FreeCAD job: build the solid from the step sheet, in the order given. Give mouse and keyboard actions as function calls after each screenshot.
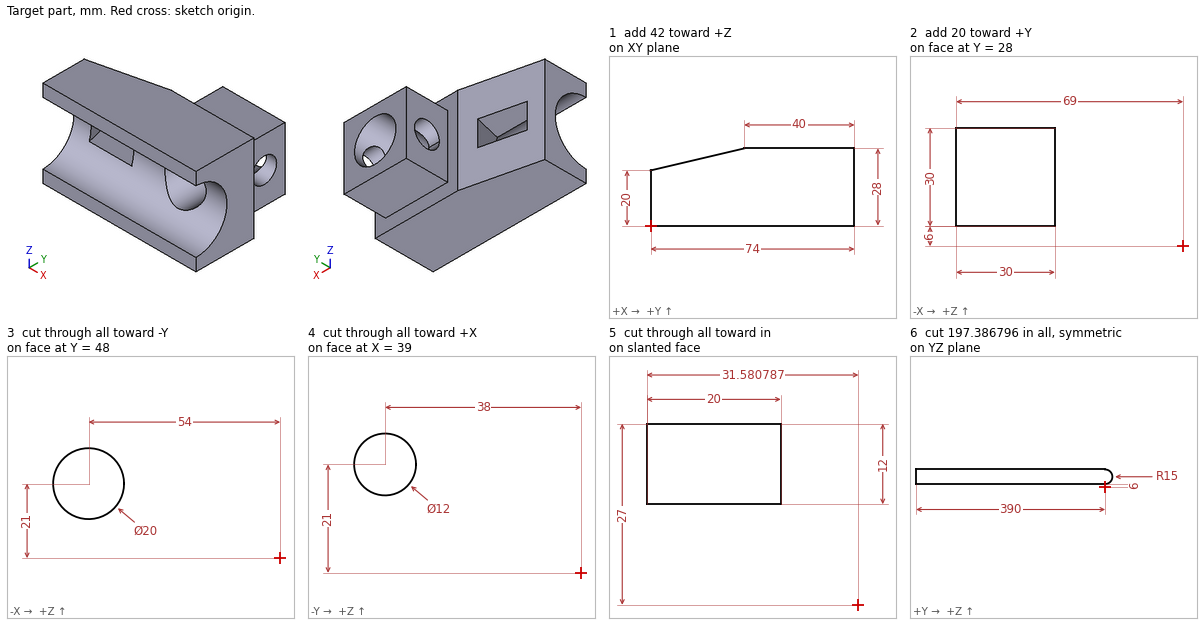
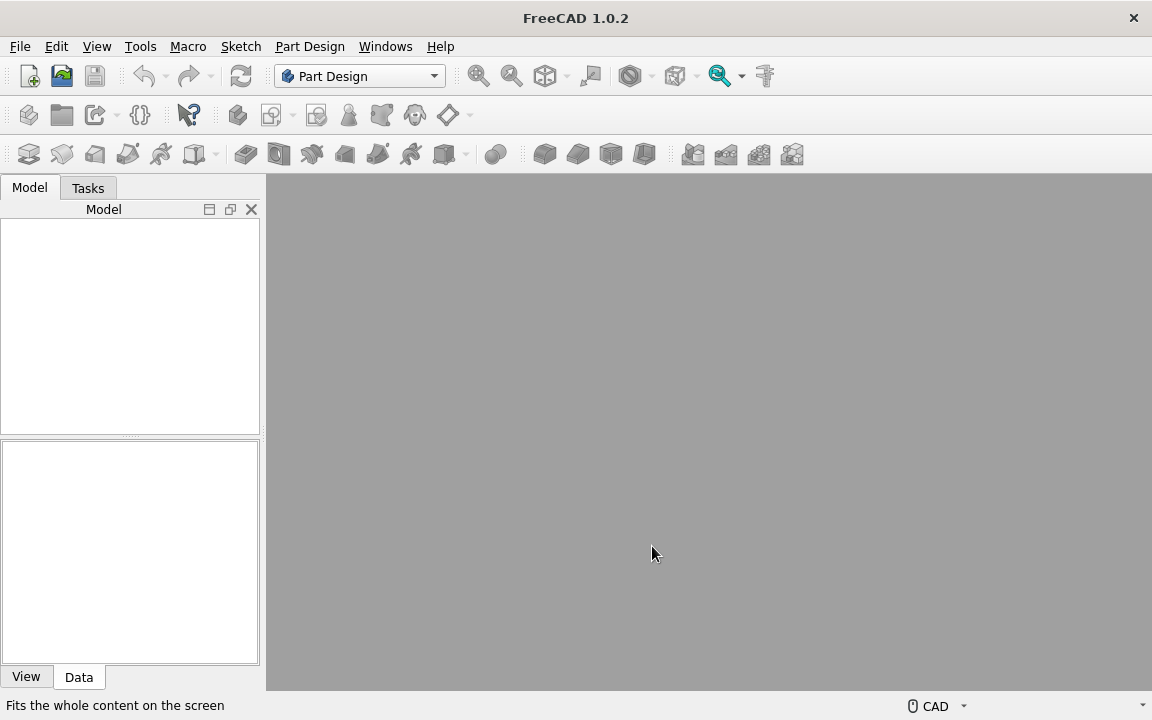
click(29, 76)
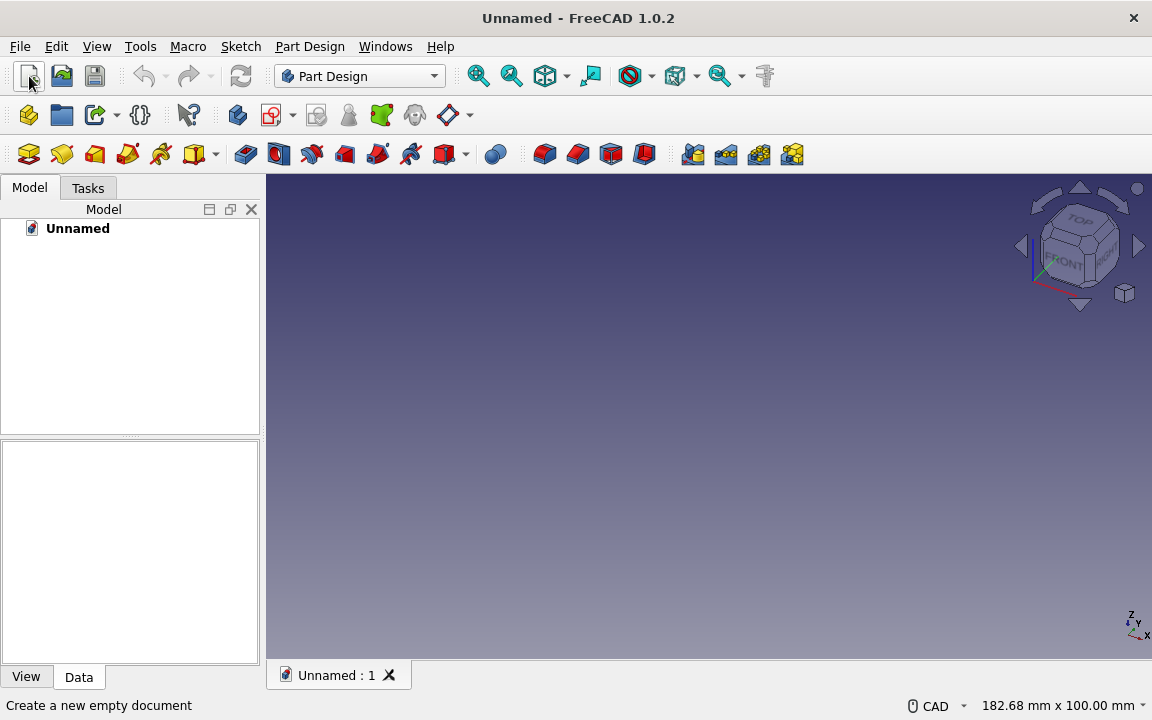
click(270, 116)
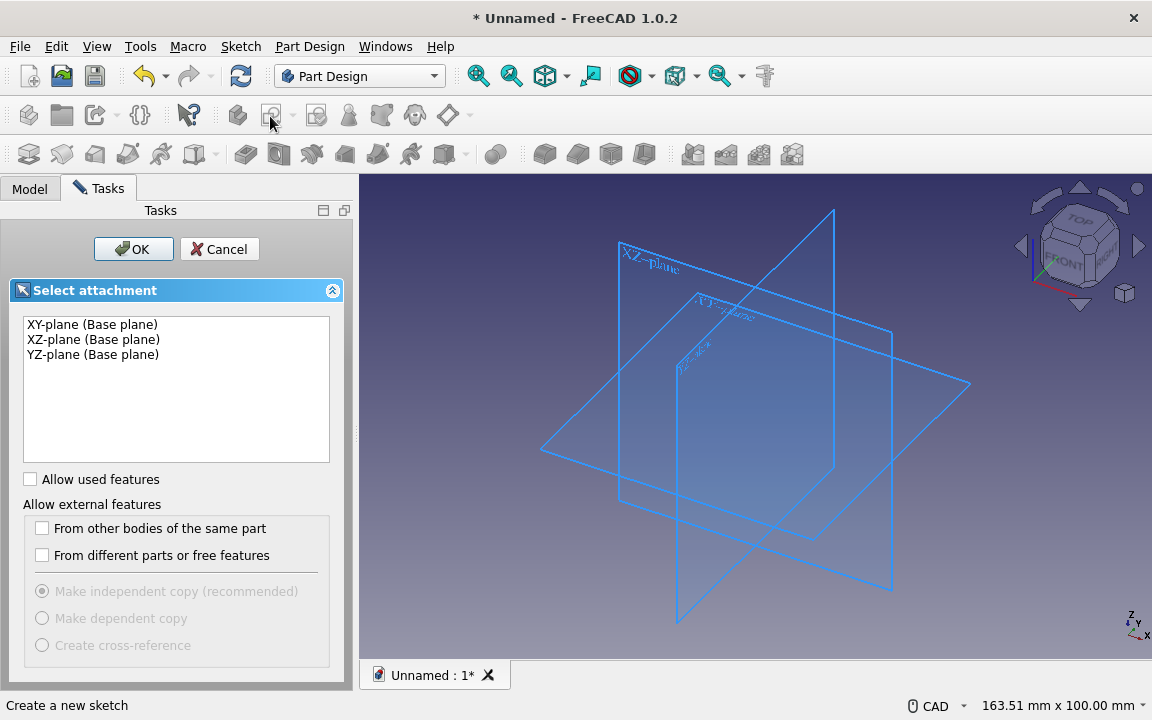
click(84, 324)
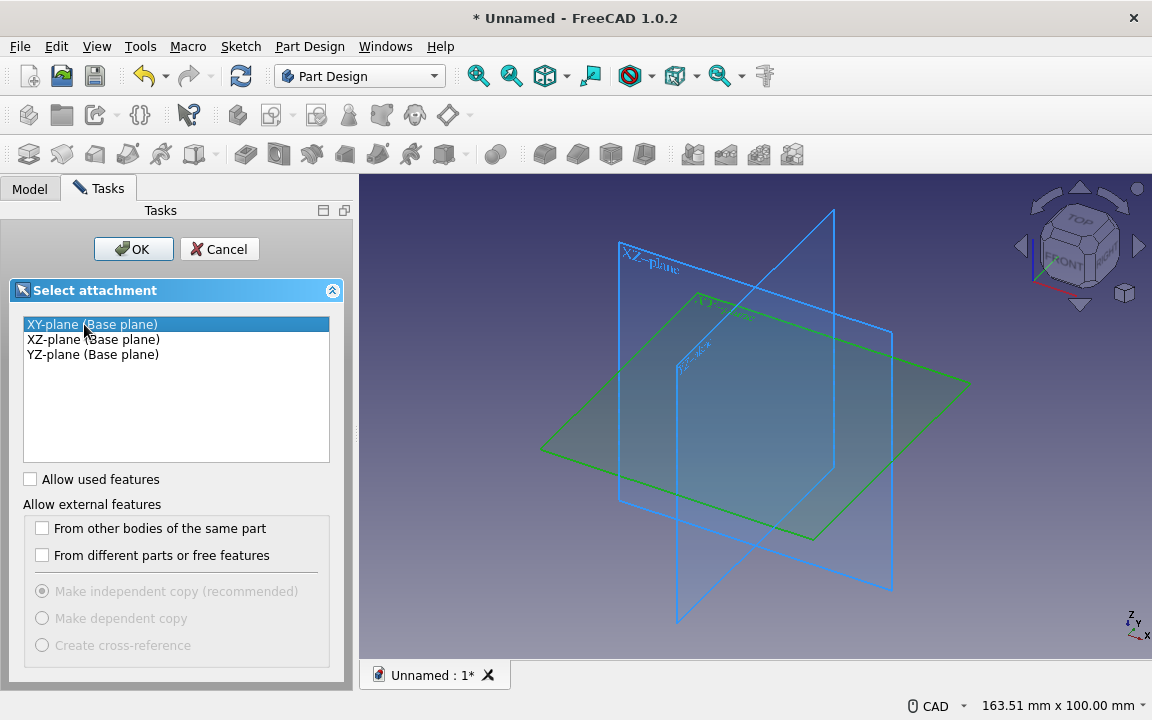
click(134, 249)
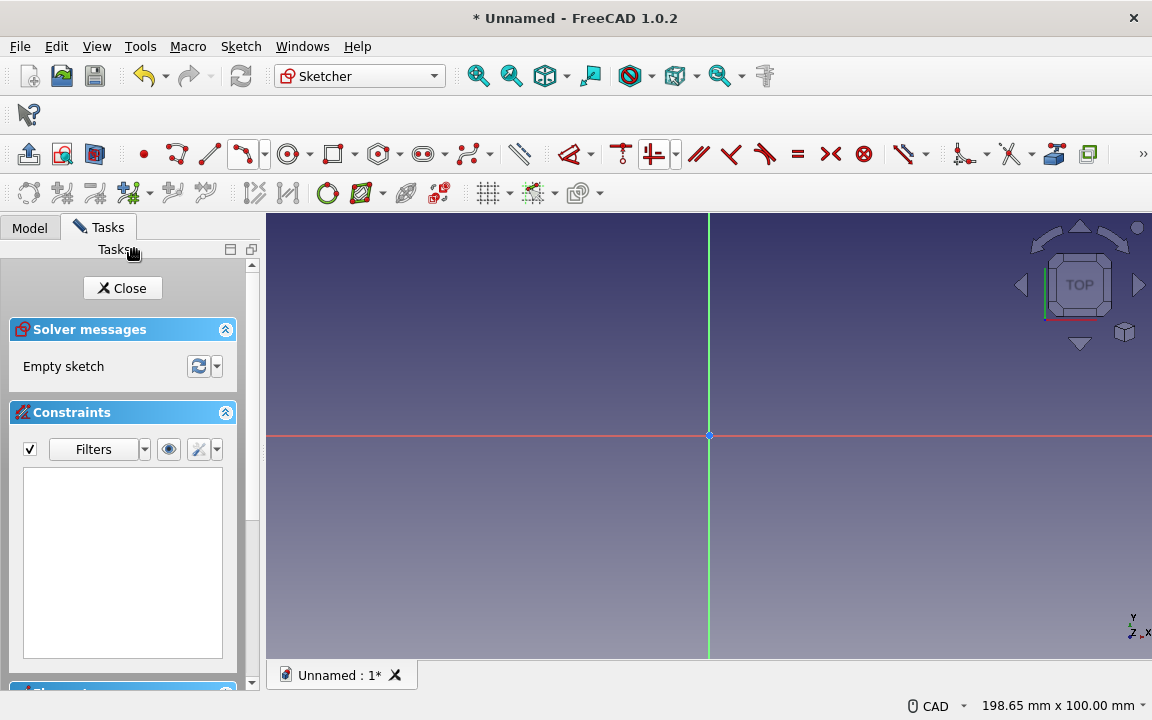
scroll(294, 631, down, 1)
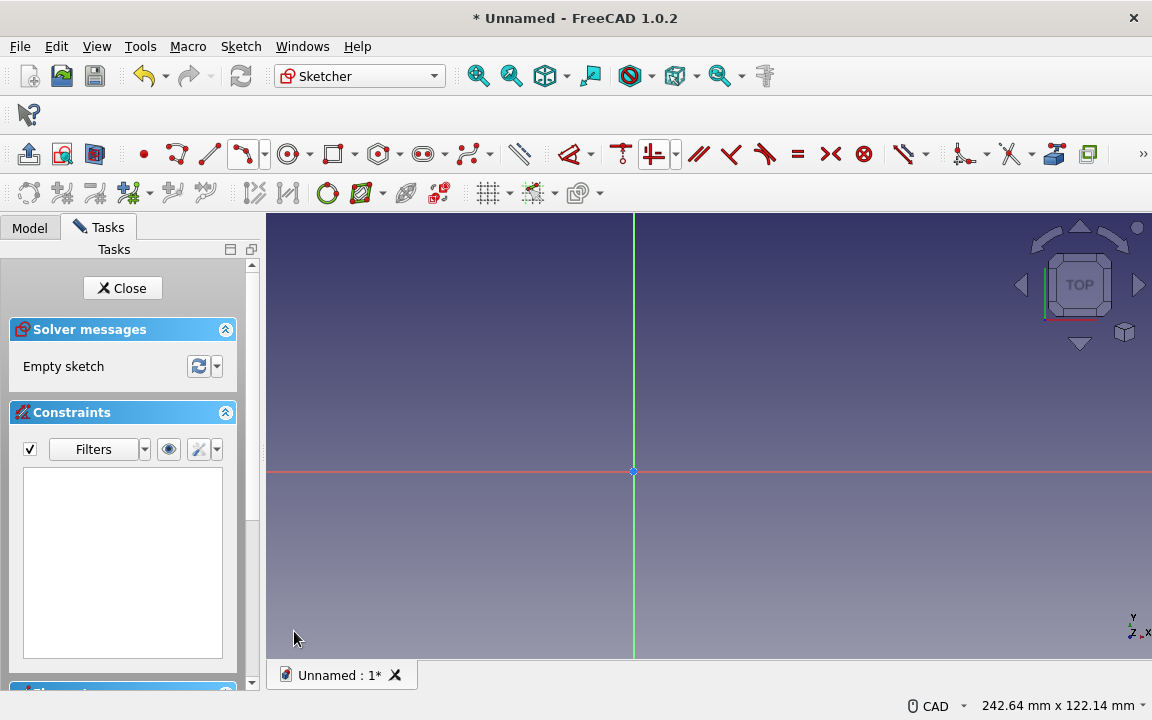
scroll(925, 401, up, 3)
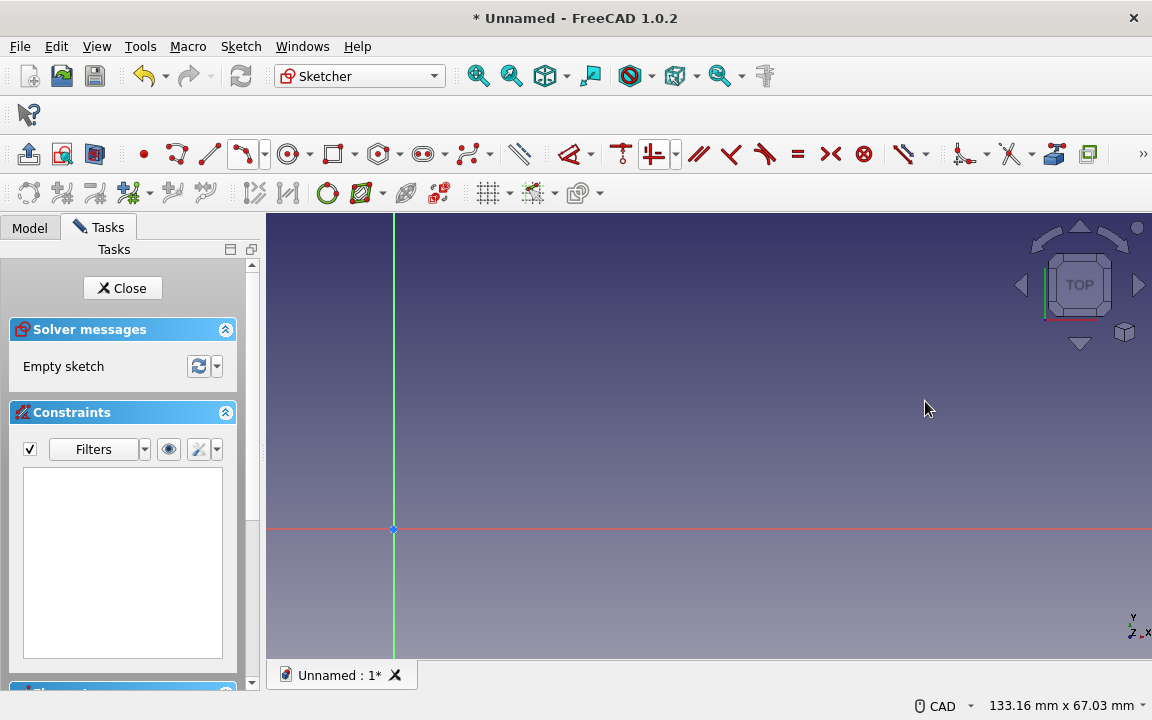
click(177, 154)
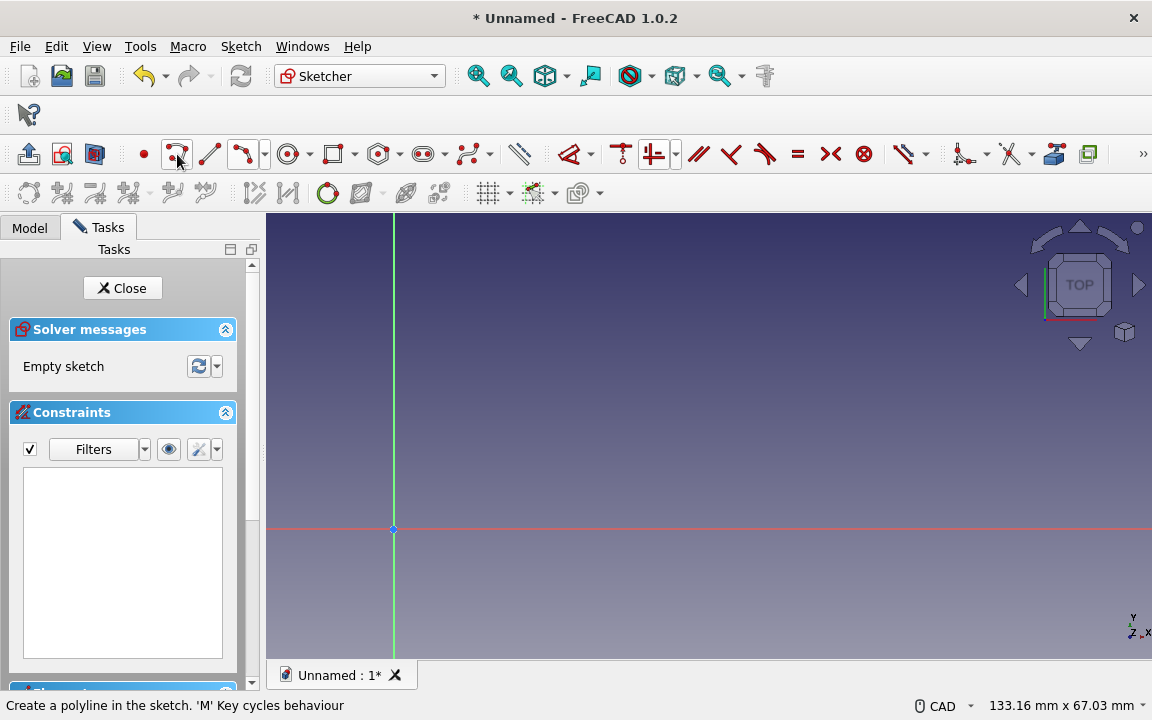
click(394, 529)
click(886, 520)
click(886, 343)
click(620, 343)
click(403, 396)
click(394, 529)
key(Escape)
key(Escape)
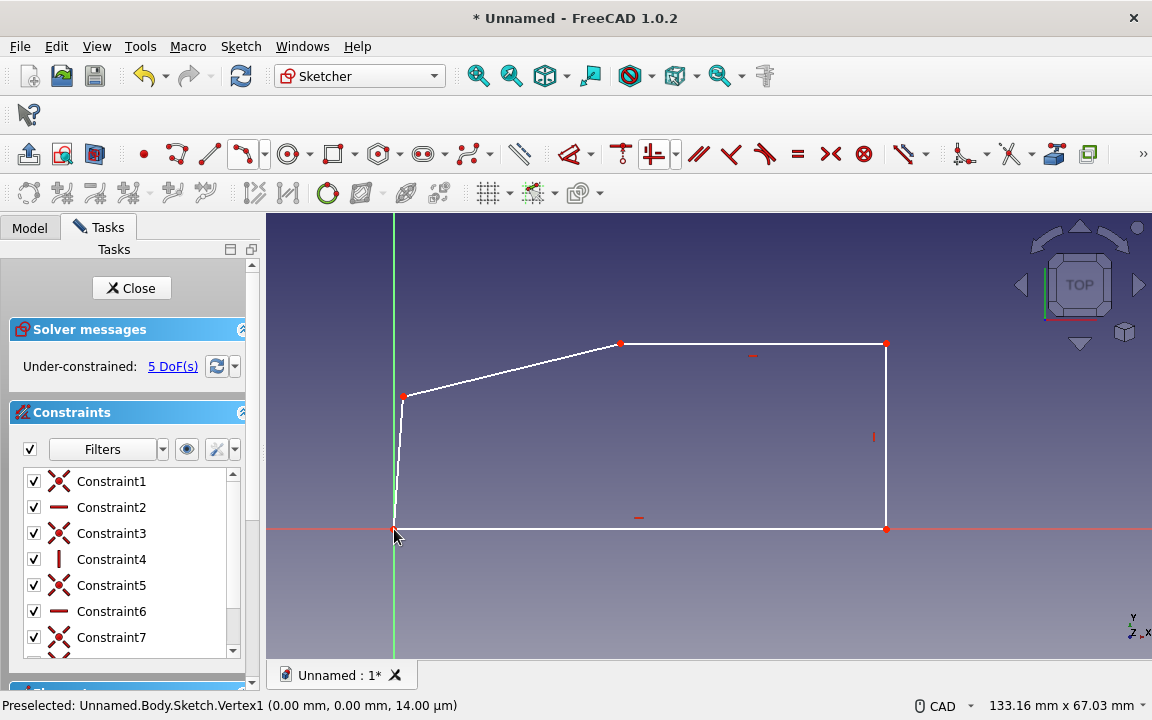
click(397, 490)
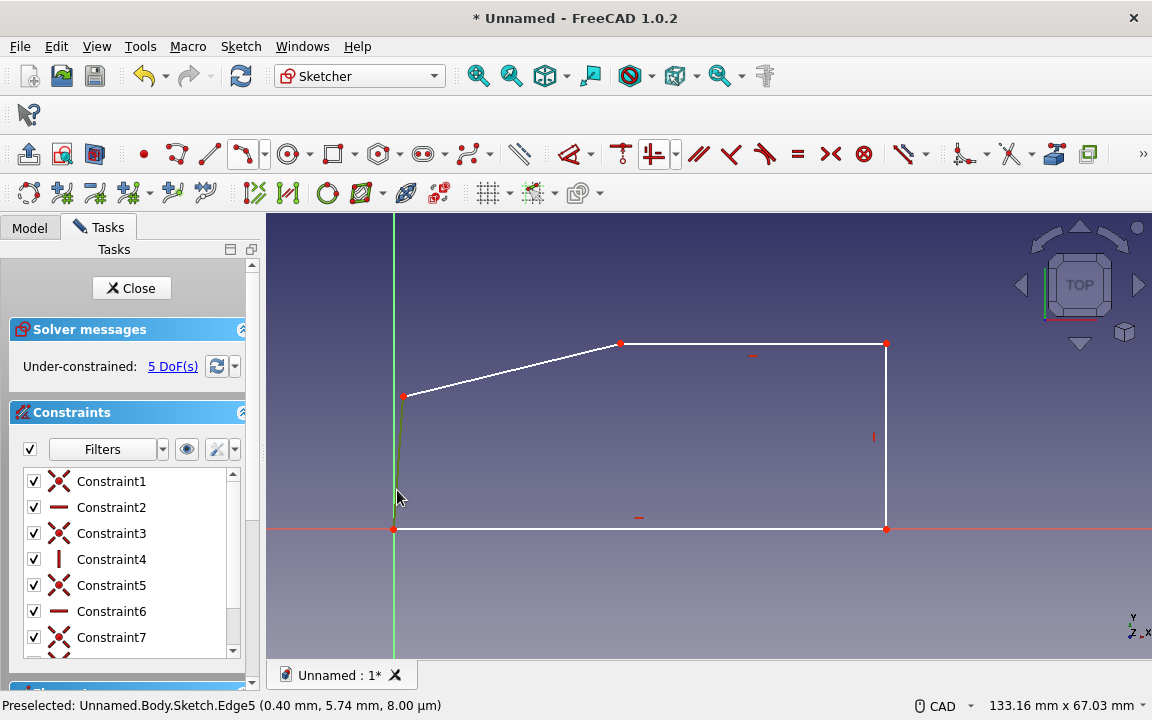
key(v)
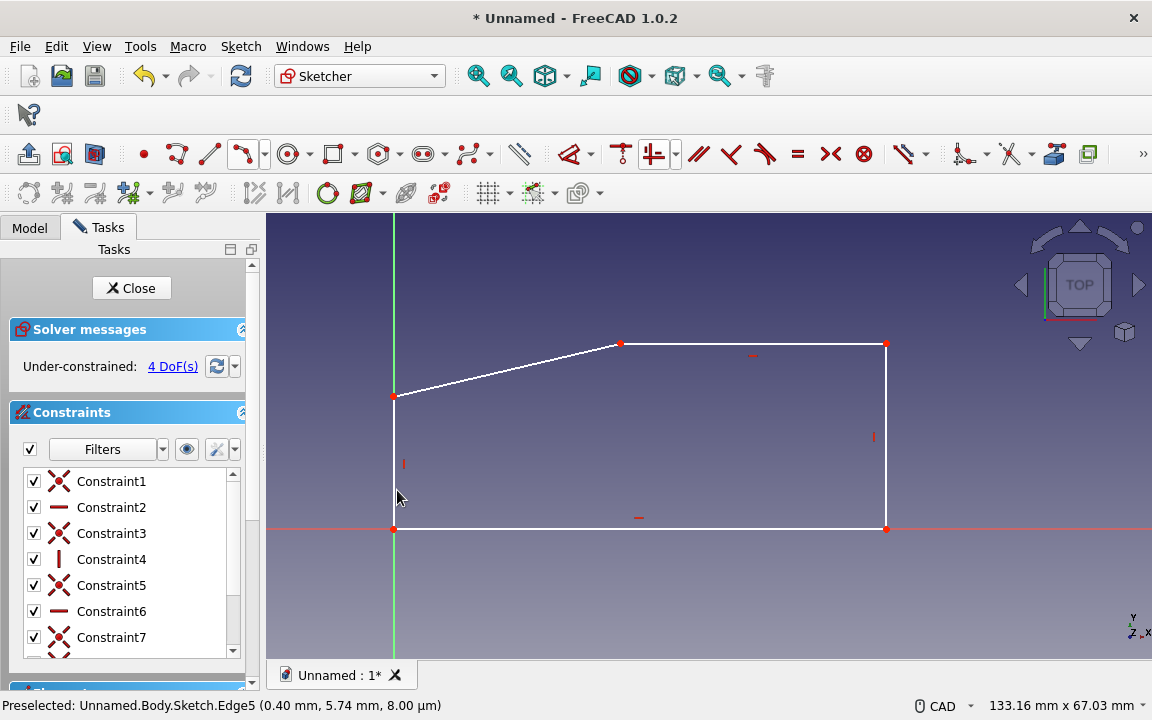
click(568, 154)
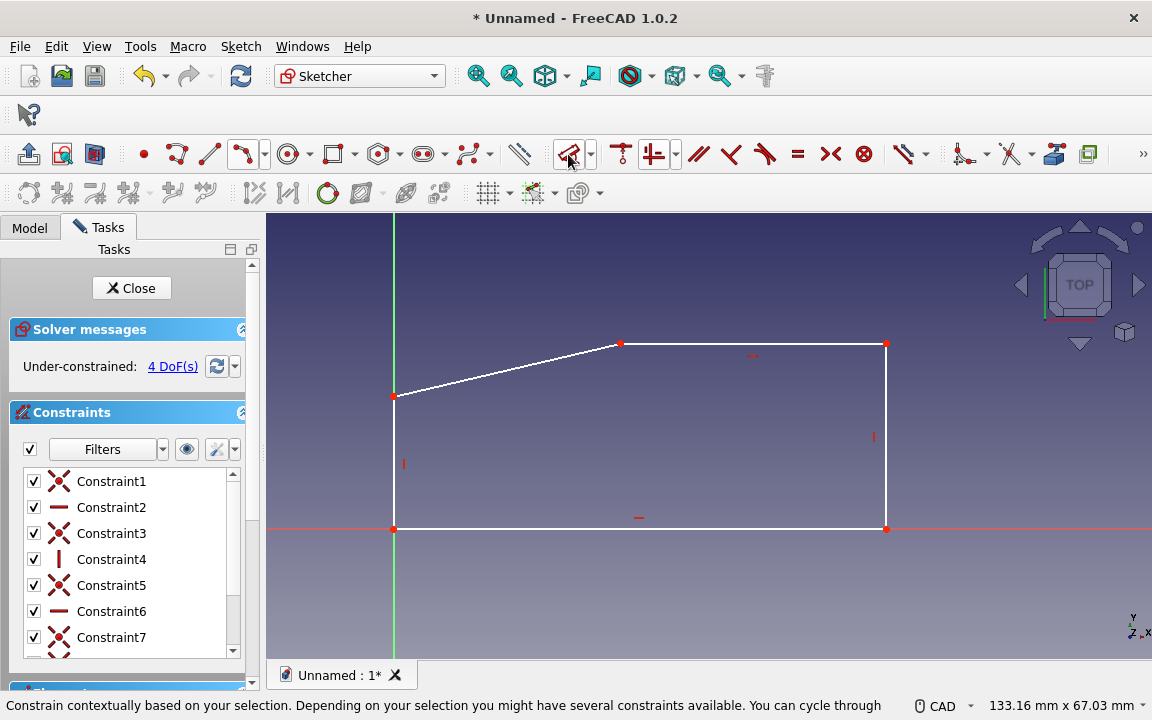
click(541, 529)
click(640, 563)